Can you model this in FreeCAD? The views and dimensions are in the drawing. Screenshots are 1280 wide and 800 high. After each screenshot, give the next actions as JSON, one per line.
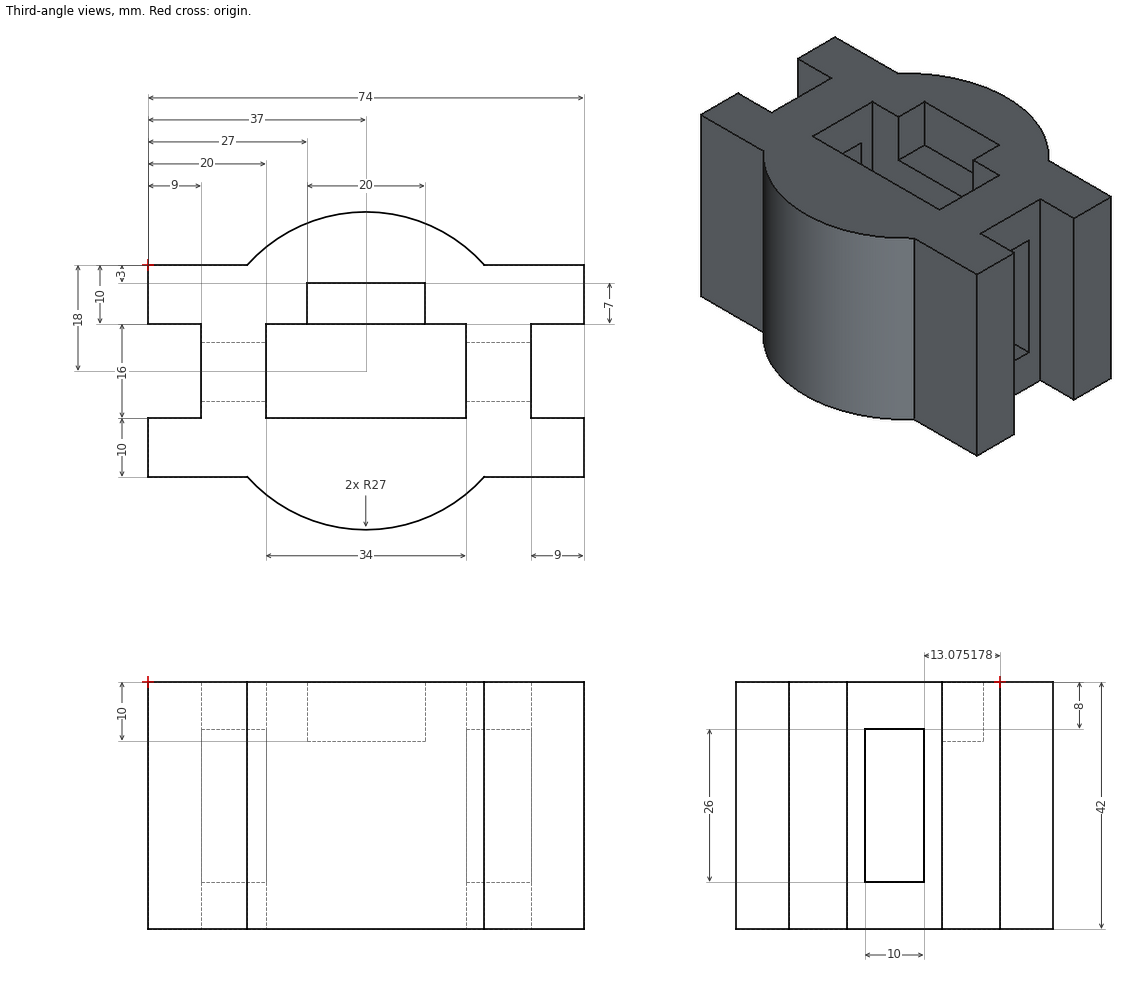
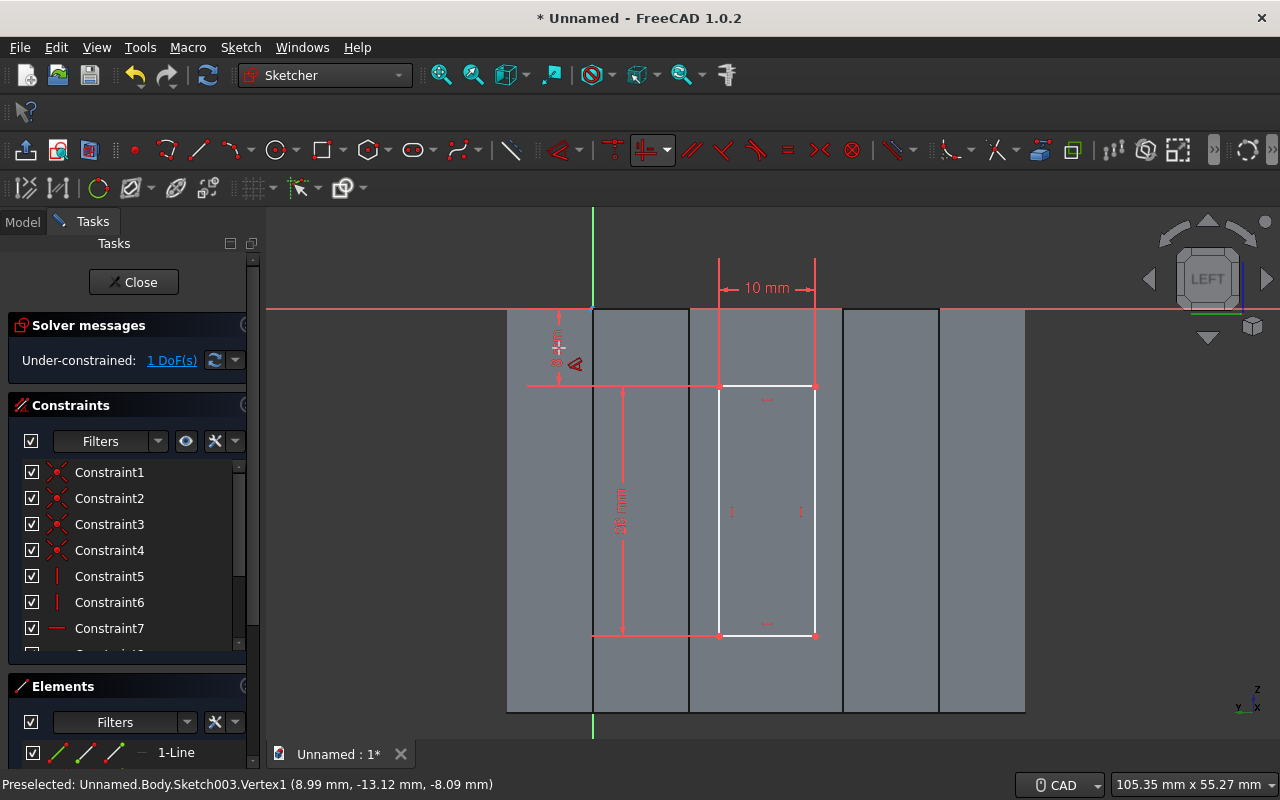
{"action": "left_click", "coordinate": [719, 386]}
{"action": "left_click", "coordinate": [656, 275]}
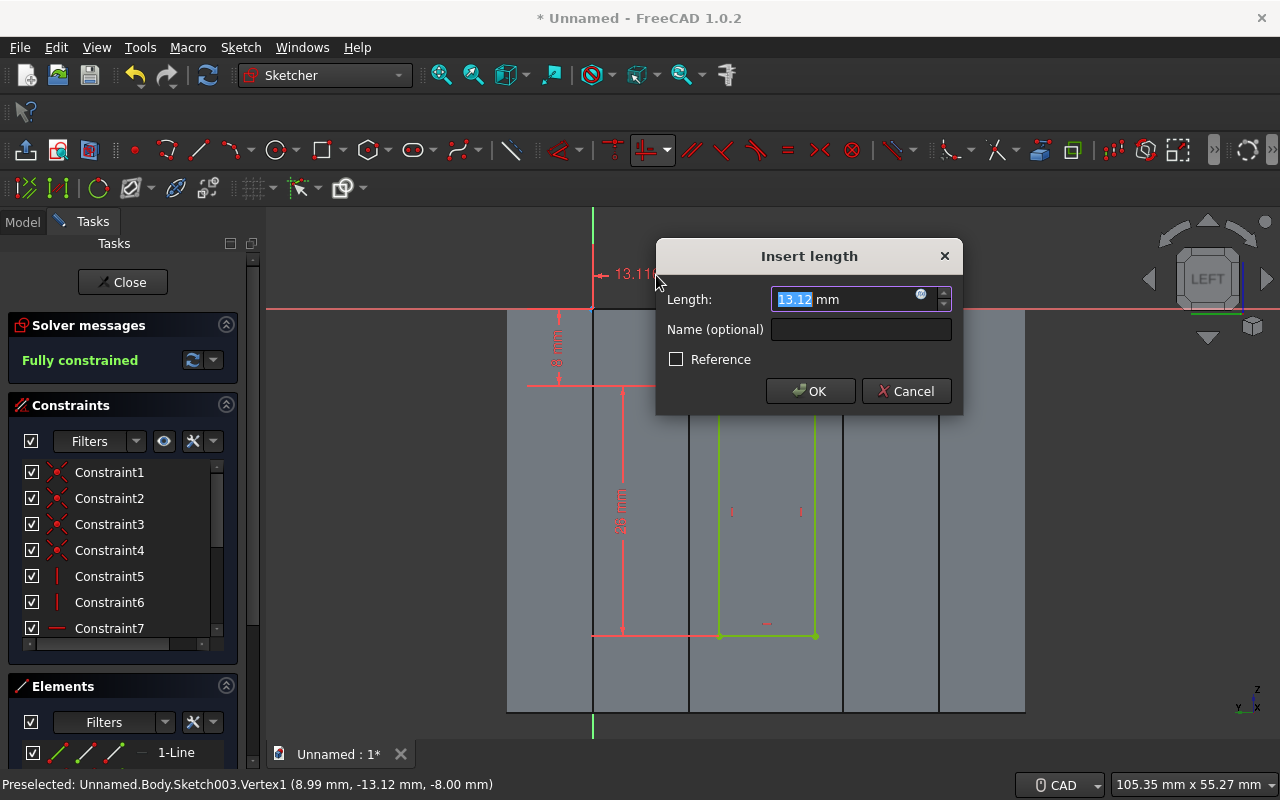
{"action": "type", "text": "13.075178"}
{"action": "key", "text": "Return"}
{"action": "key", "text": "Escape"}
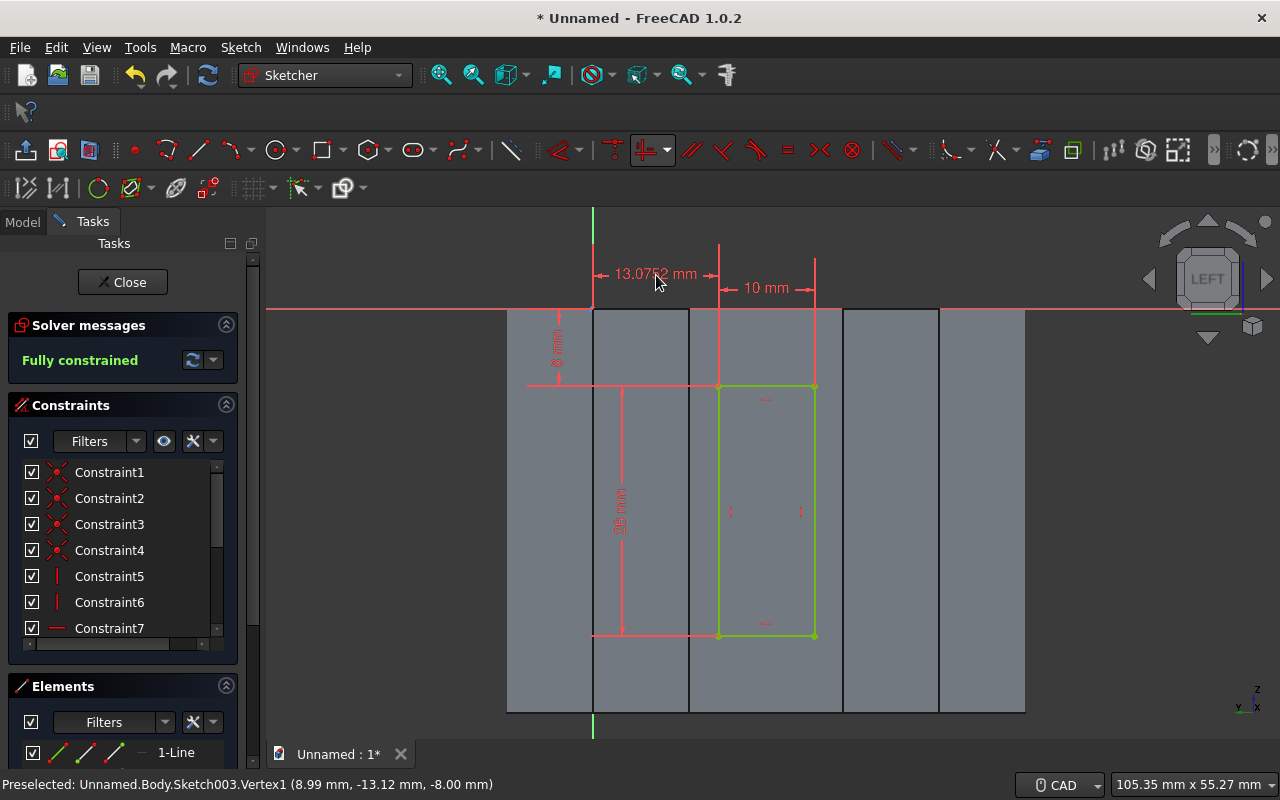
{"action": "left_click", "coordinate": [123, 282]}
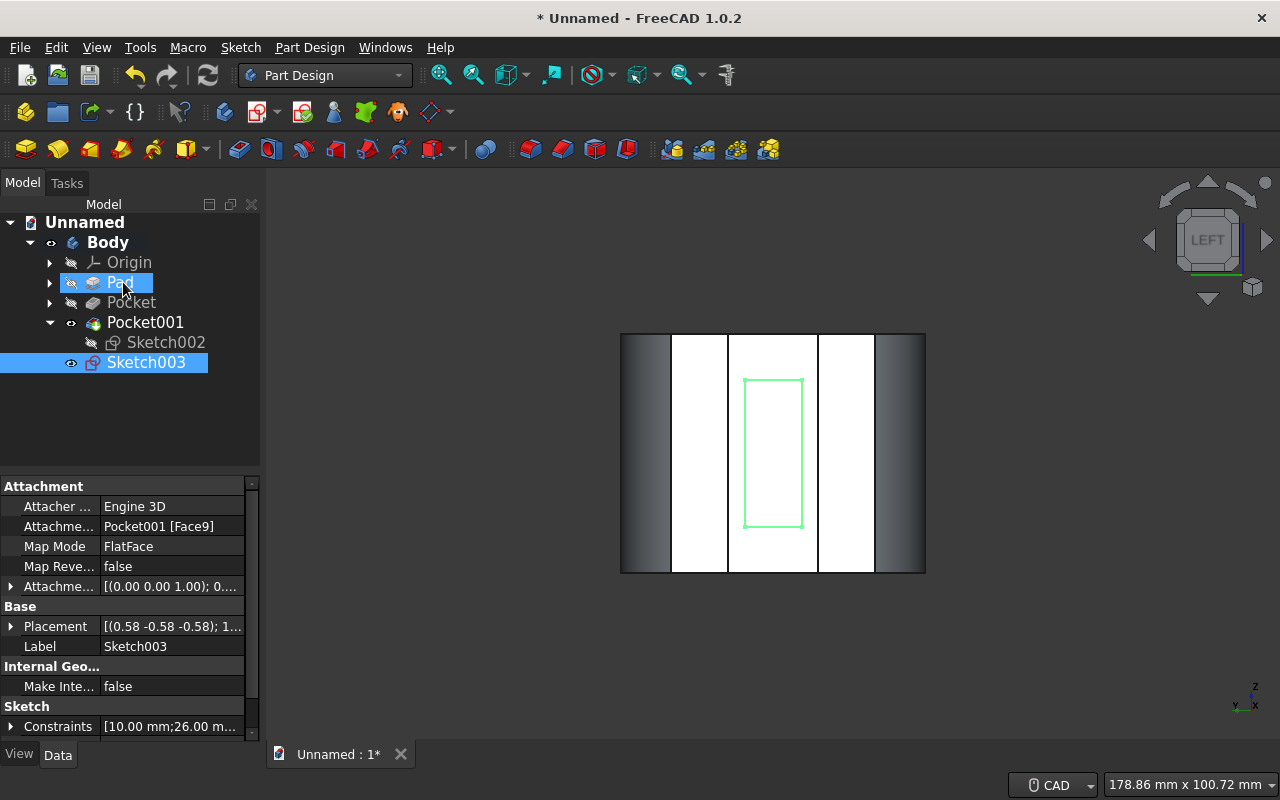
{"action": "left_click", "coordinate": [240, 150]}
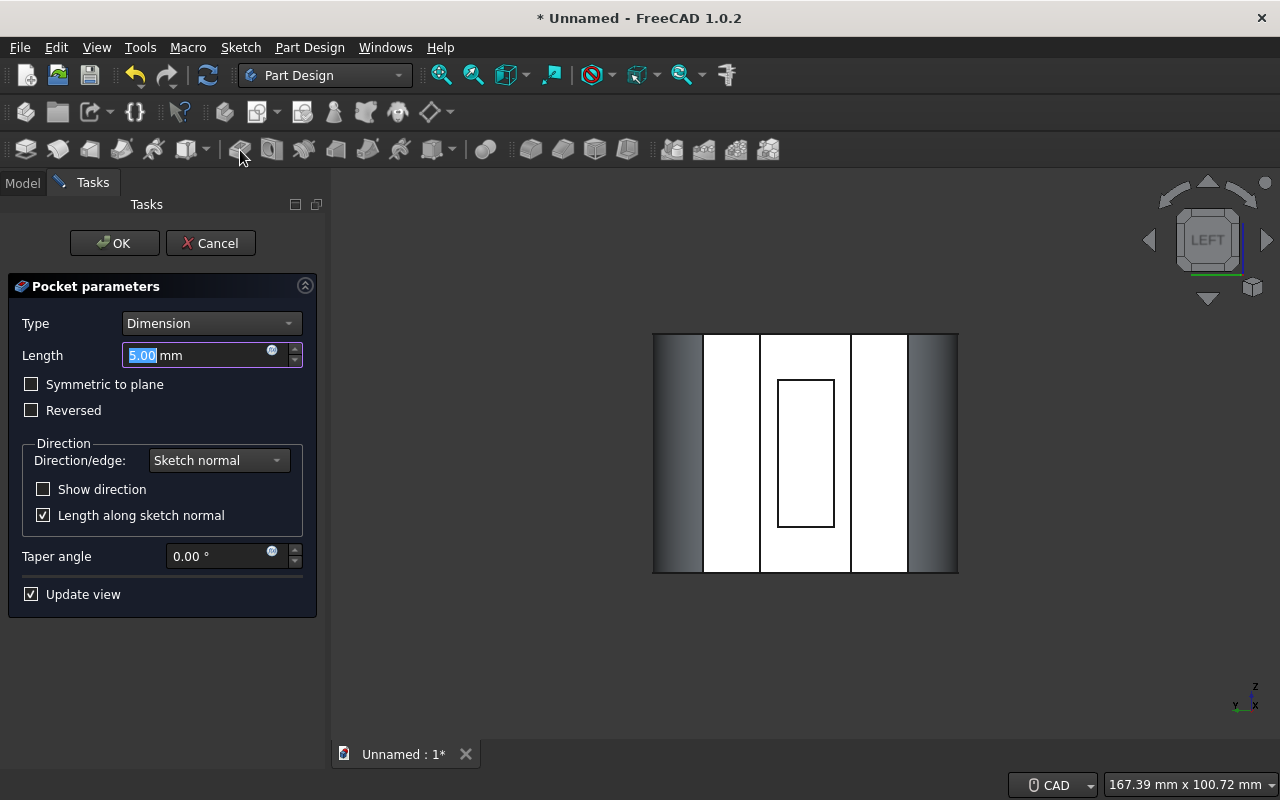
{"action": "left_click", "coordinate": [212, 324]}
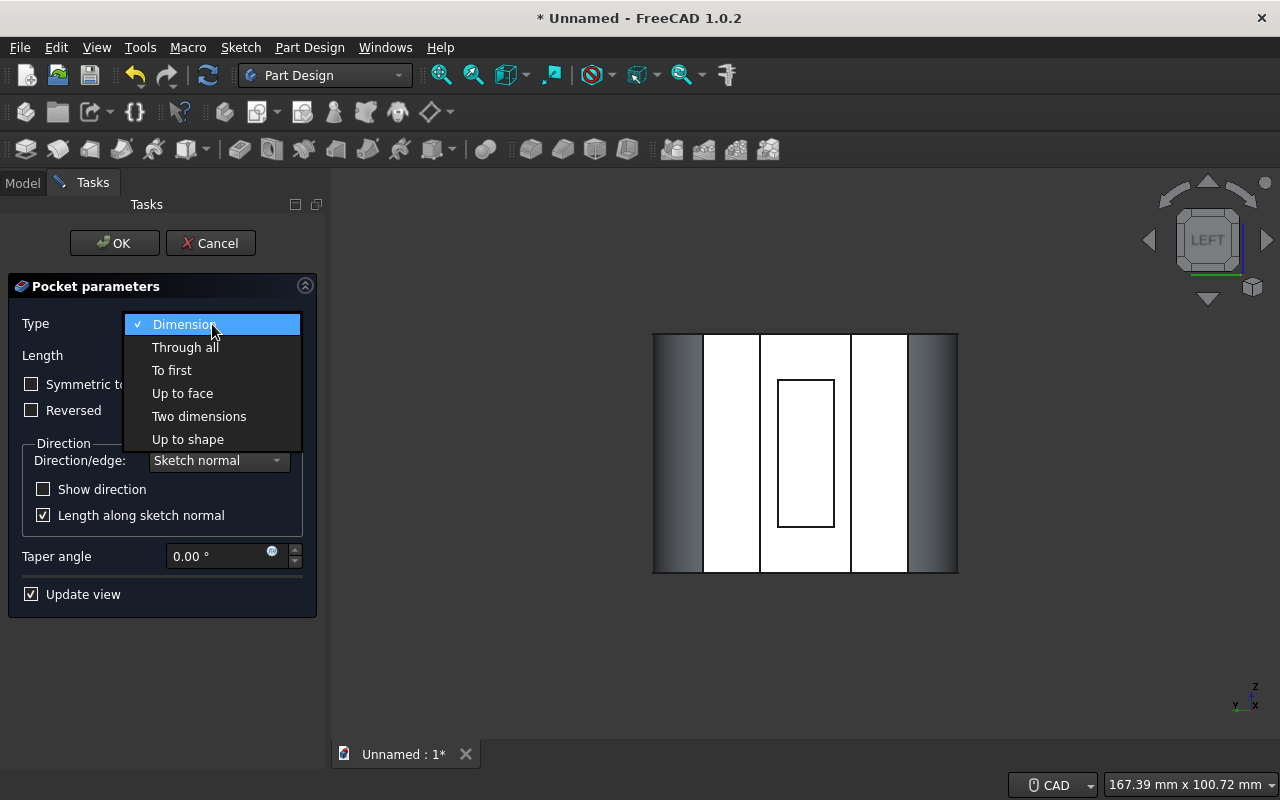
{"action": "left_click", "coordinate": [212, 348]}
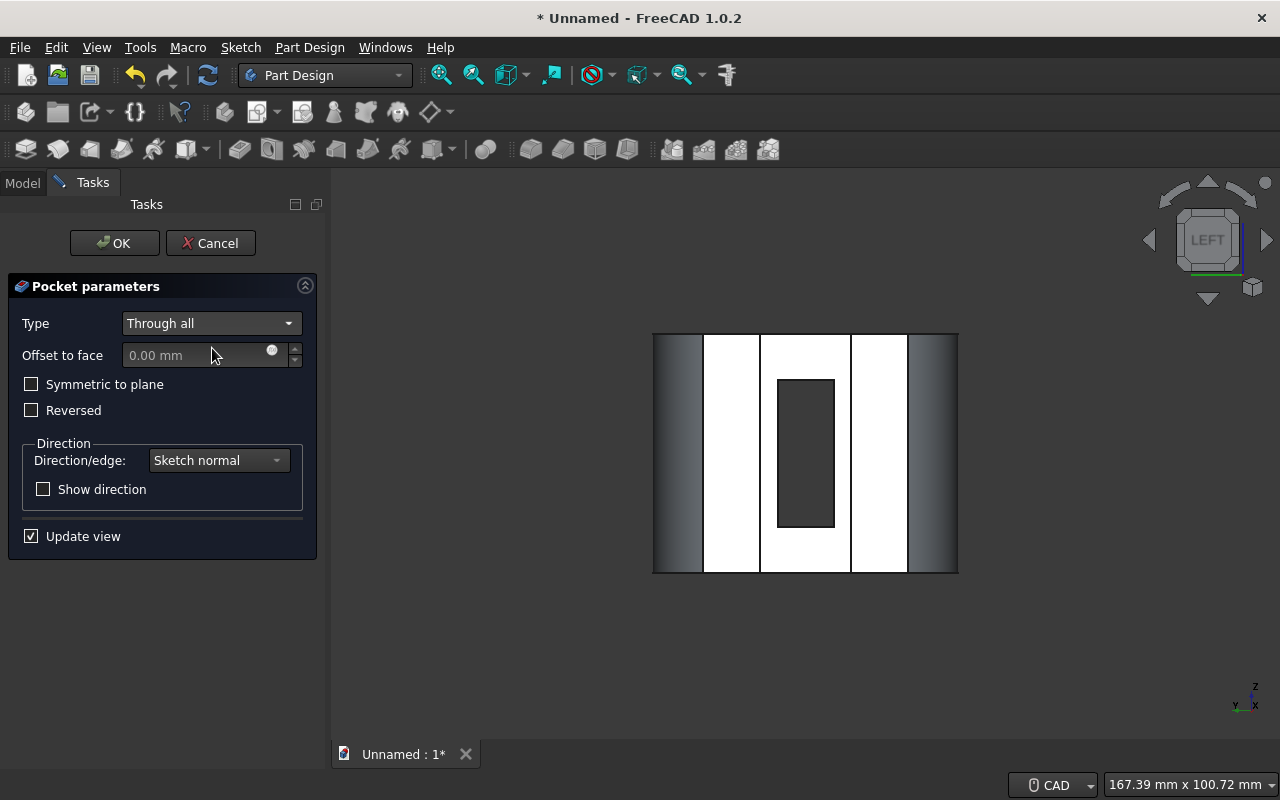
{"action": "left_click", "coordinate": [115, 243]}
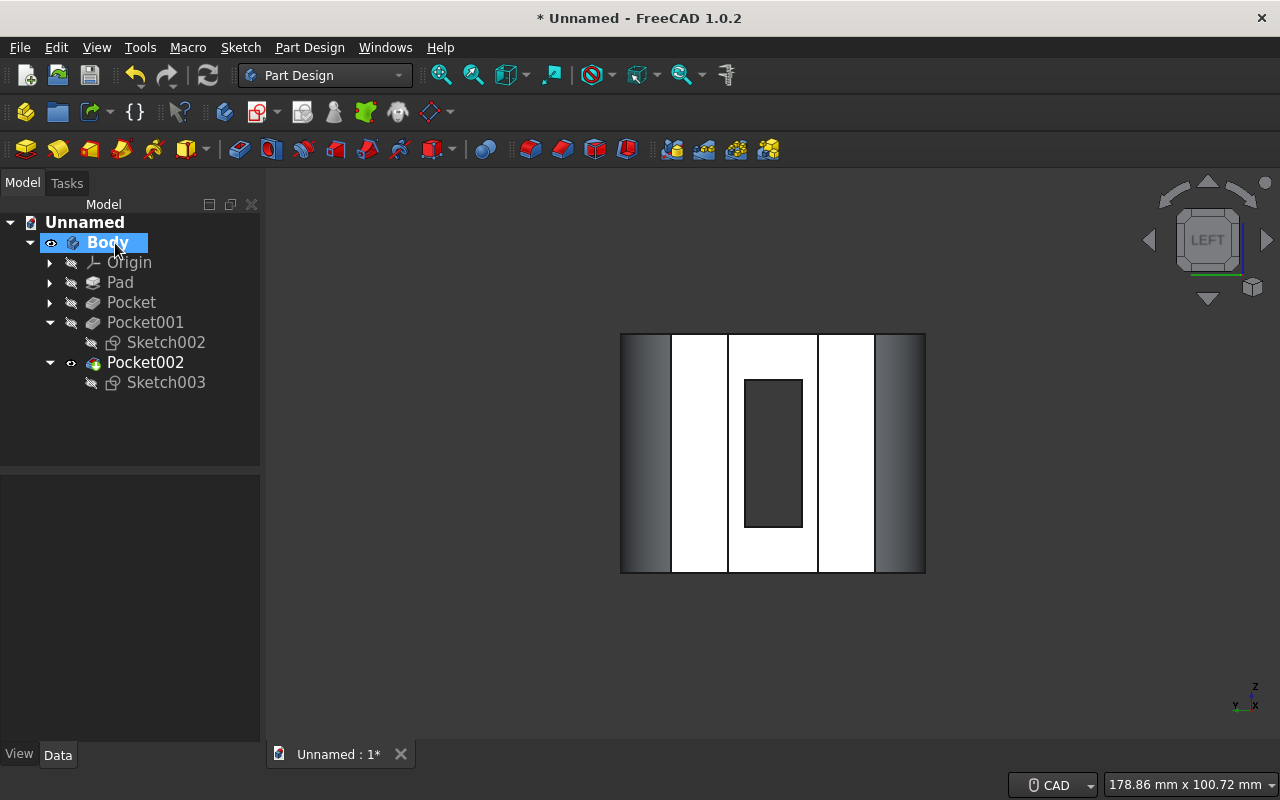
{"action": "key", "text": "0"}